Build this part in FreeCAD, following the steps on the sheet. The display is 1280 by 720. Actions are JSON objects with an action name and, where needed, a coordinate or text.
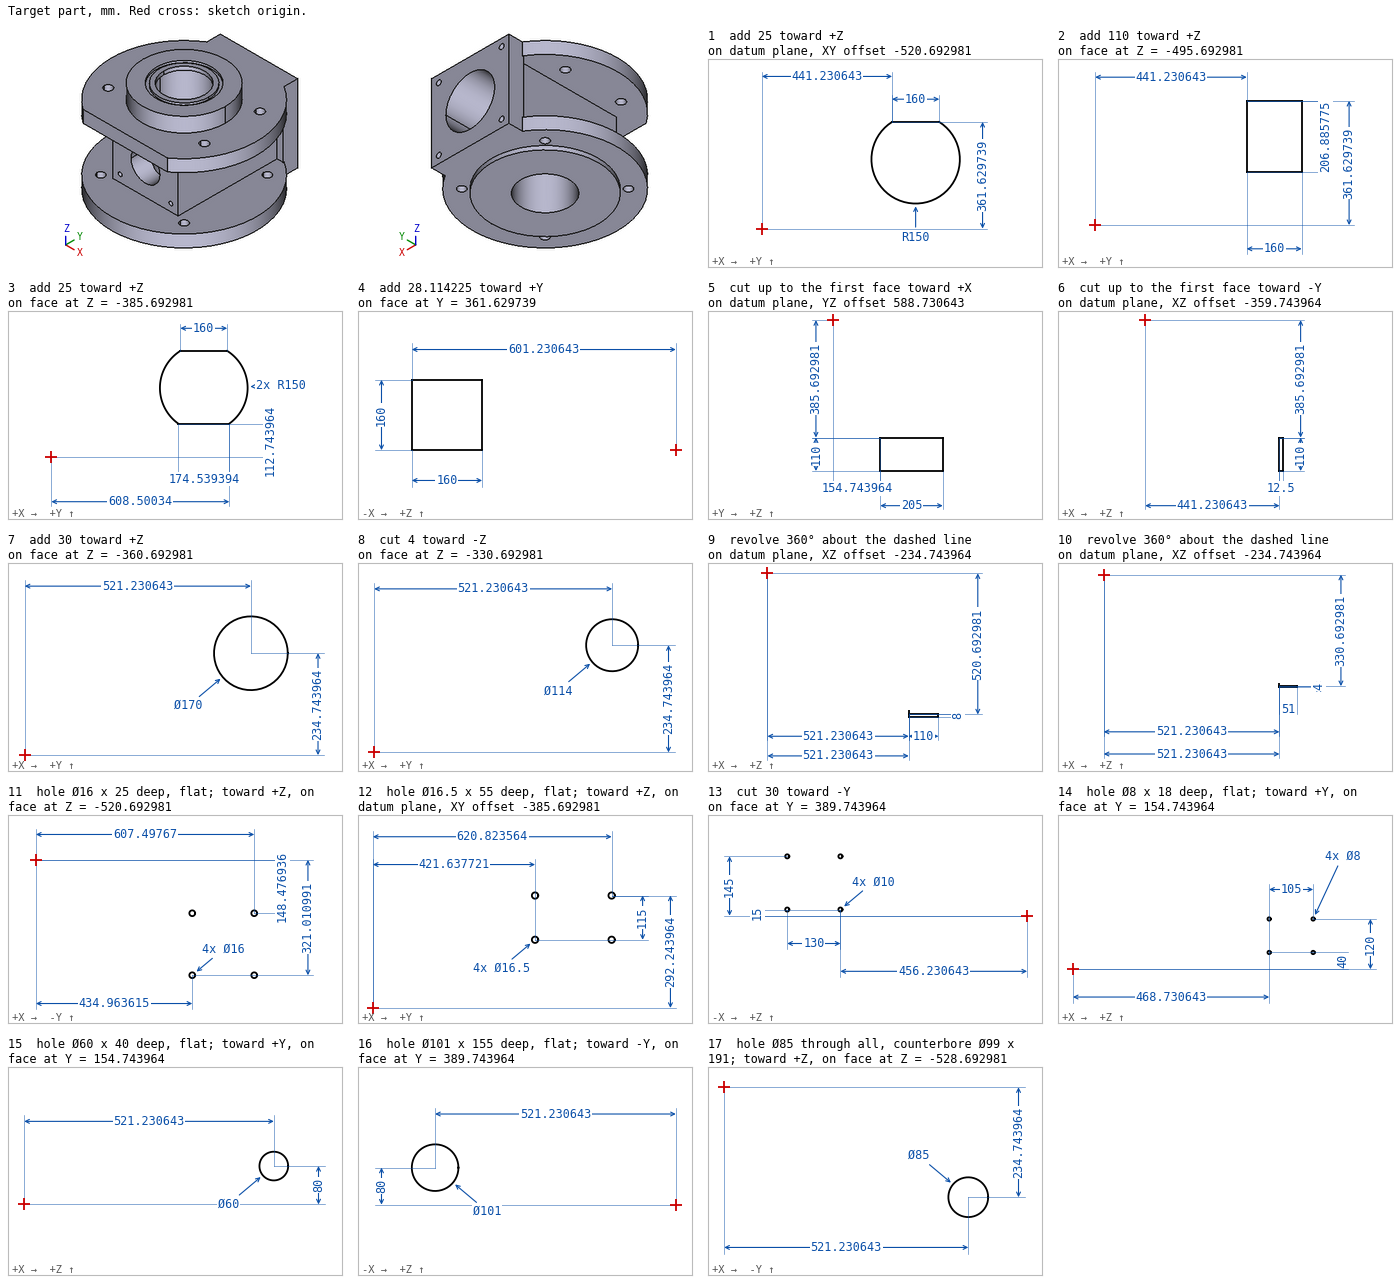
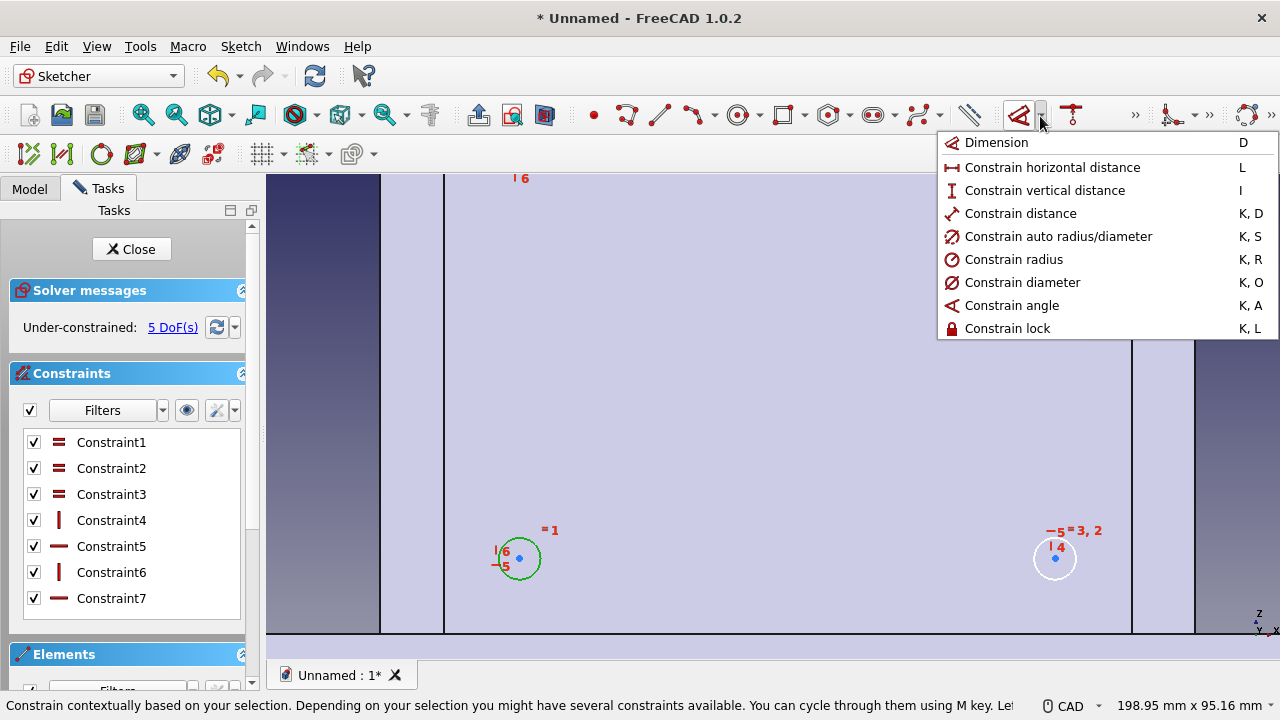
{"action": "left_click", "coordinate": [1108, 282]}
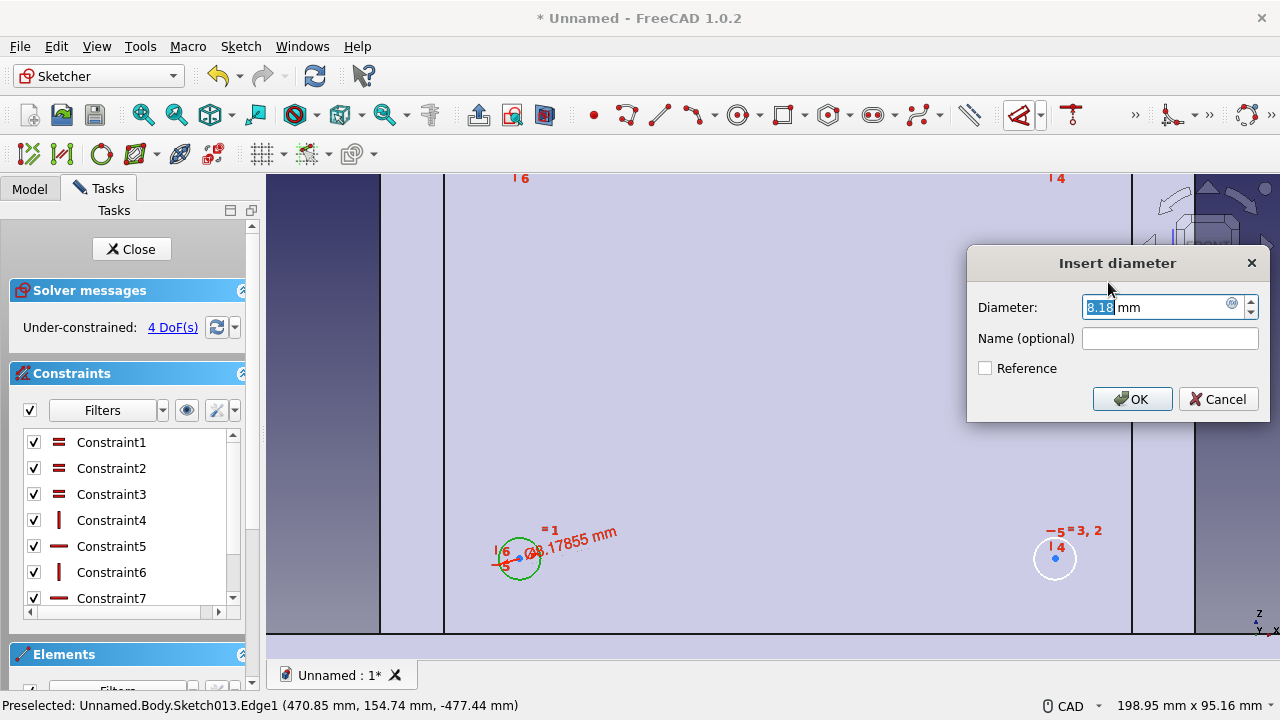
{"action": "type", "text": "8"}
{"action": "key", "text": "Return"}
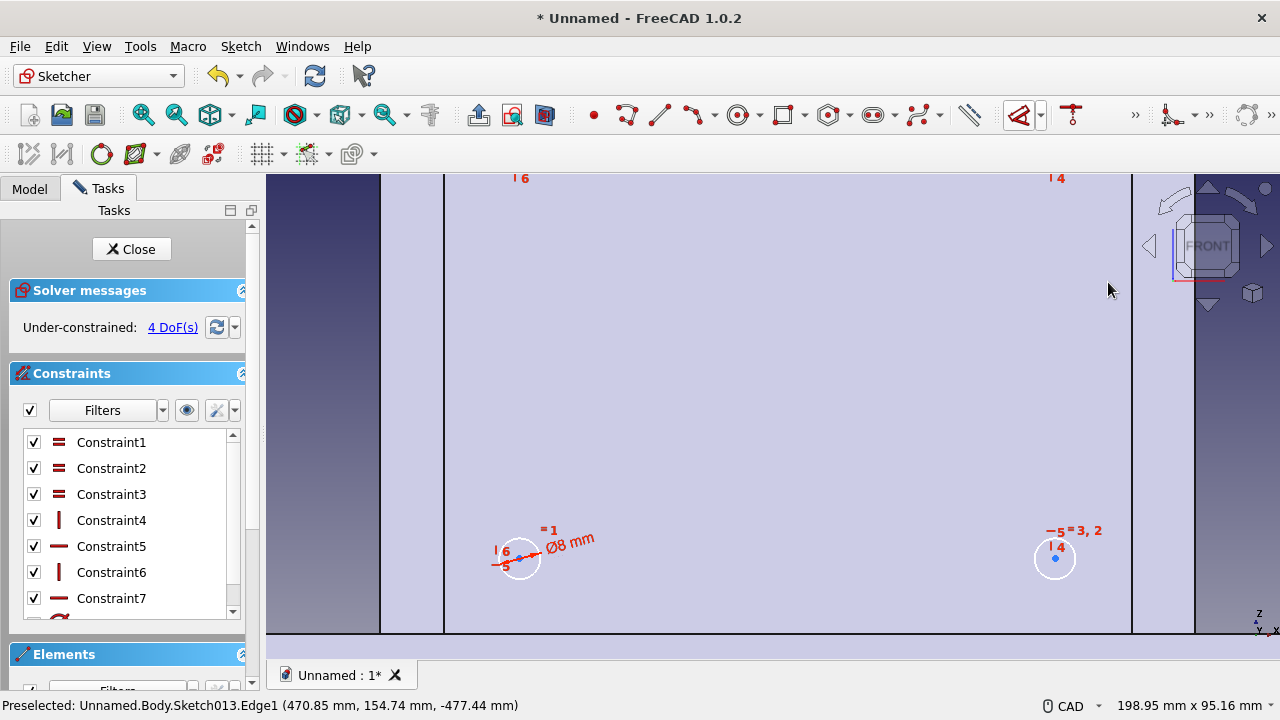
{"action": "left_click", "coordinate": [520, 559]}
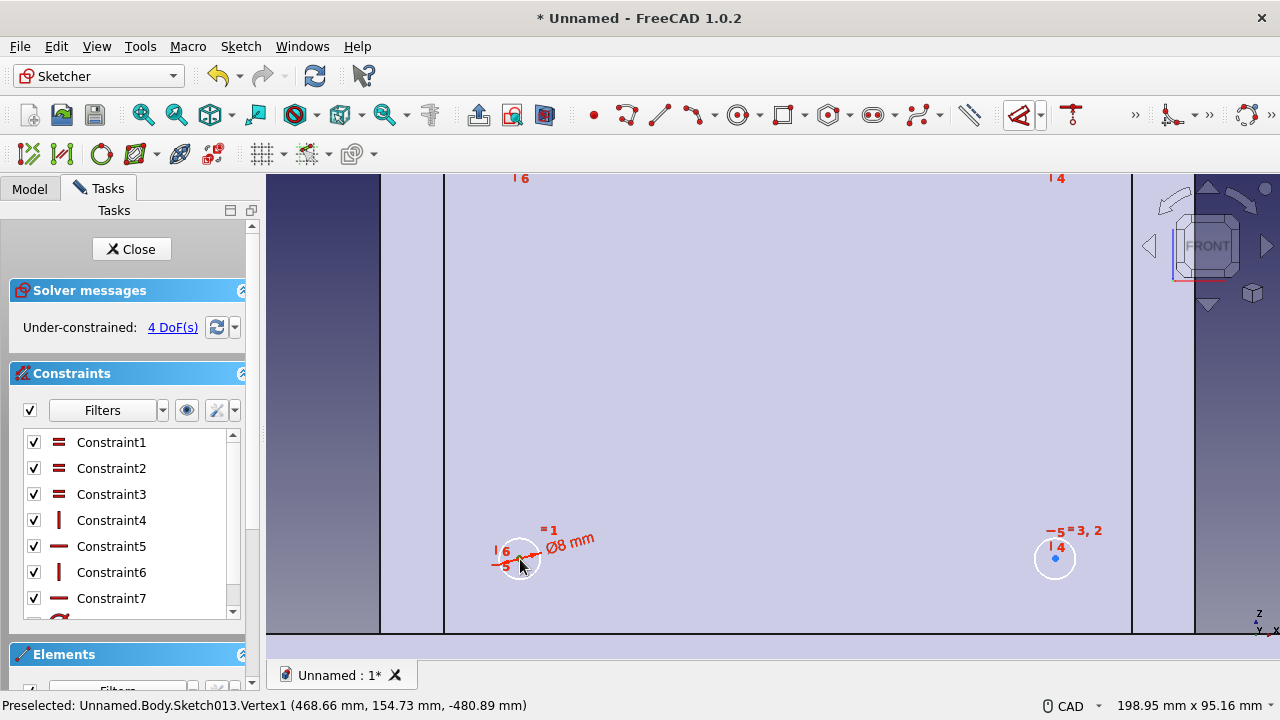
{"action": "key", "text": "i"}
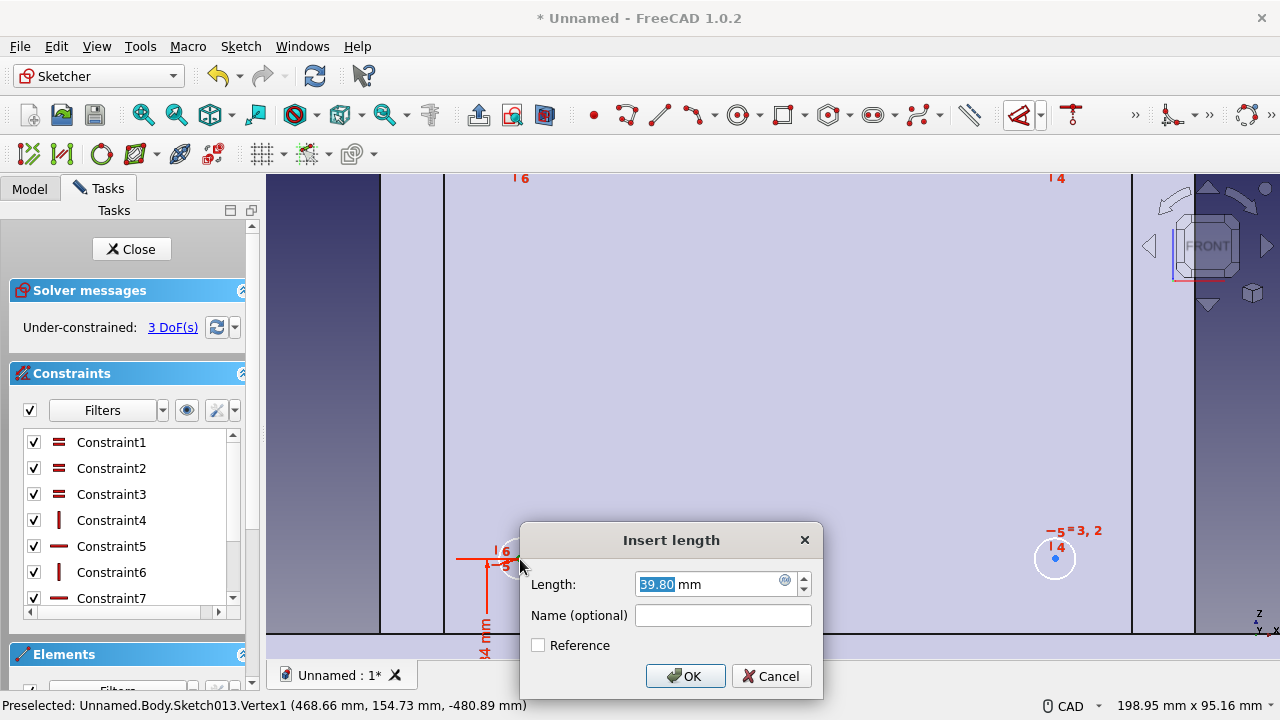
{"action": "type", "text": "40"}
{"action": "key", "text": "Return"}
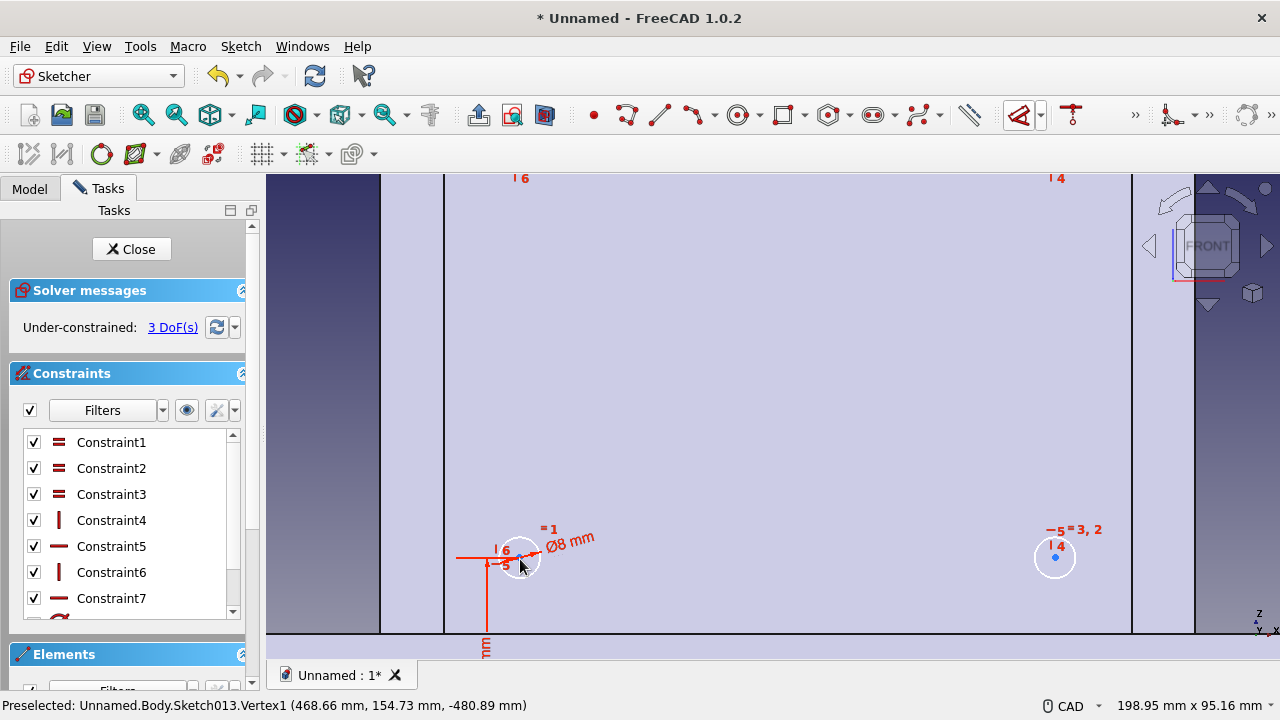
{"action": "scroll", "coordinate": [535, 544], "scroll_direction": "down", "scroll_amount": 2}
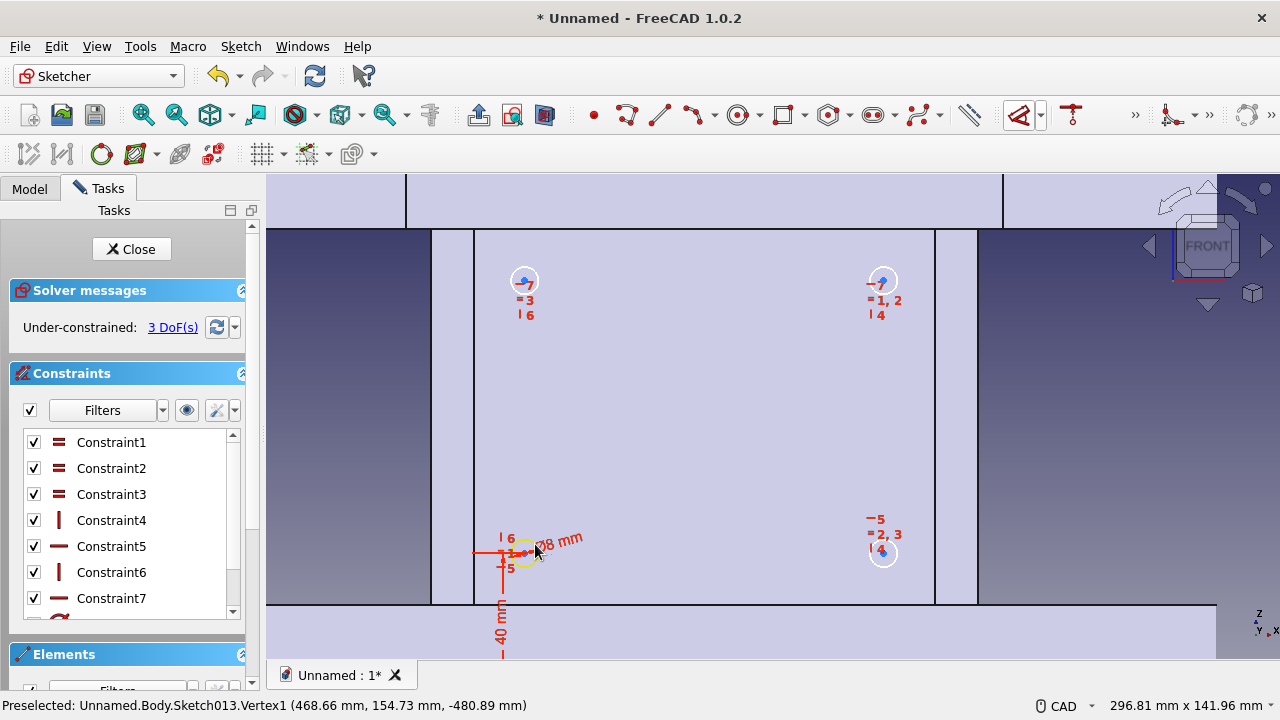
{"action": "left_click", "coordinate": [884, 281]}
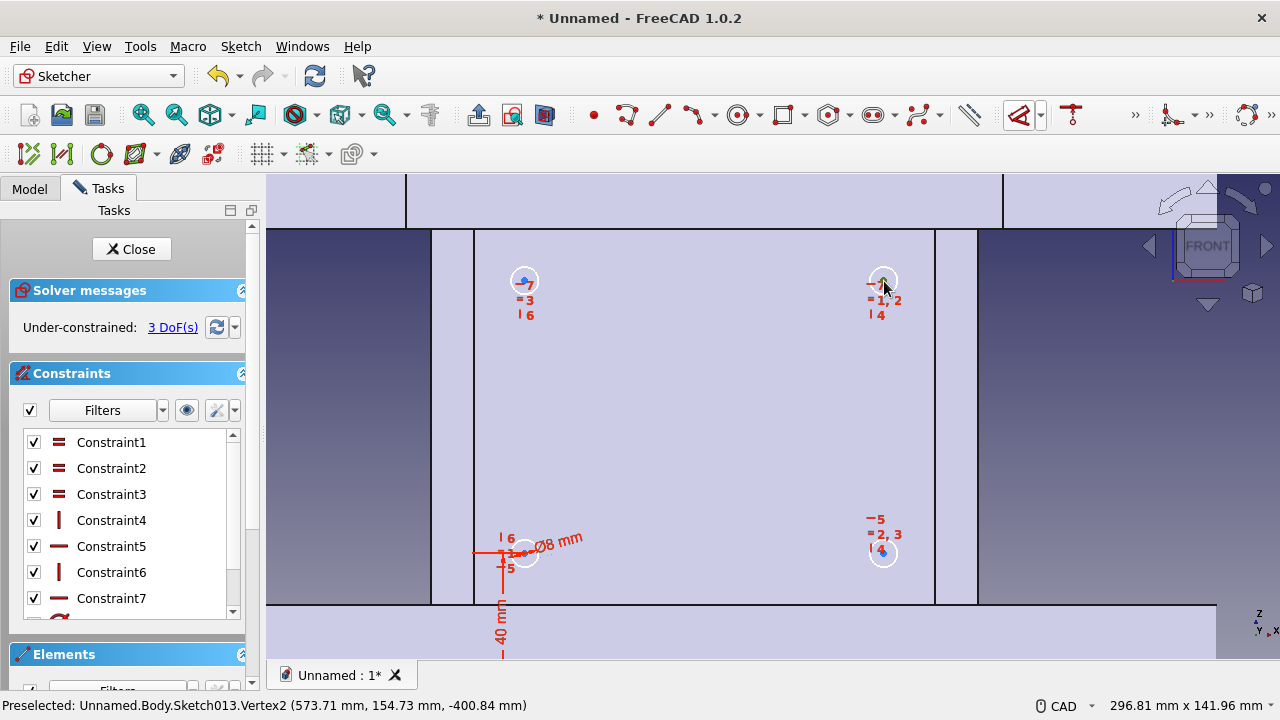
{"action": "left_click", "coordinate": [1040, 116]}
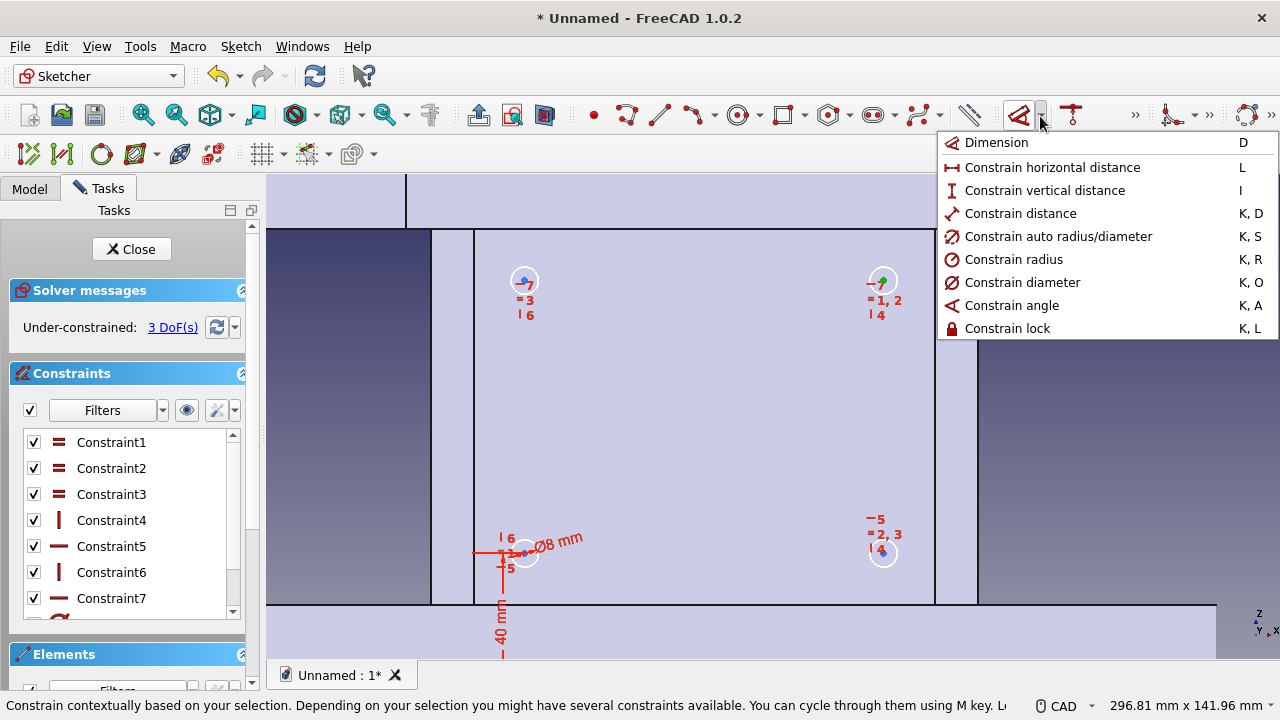
{"action": "left_click", "coordinate": [1108, 190]}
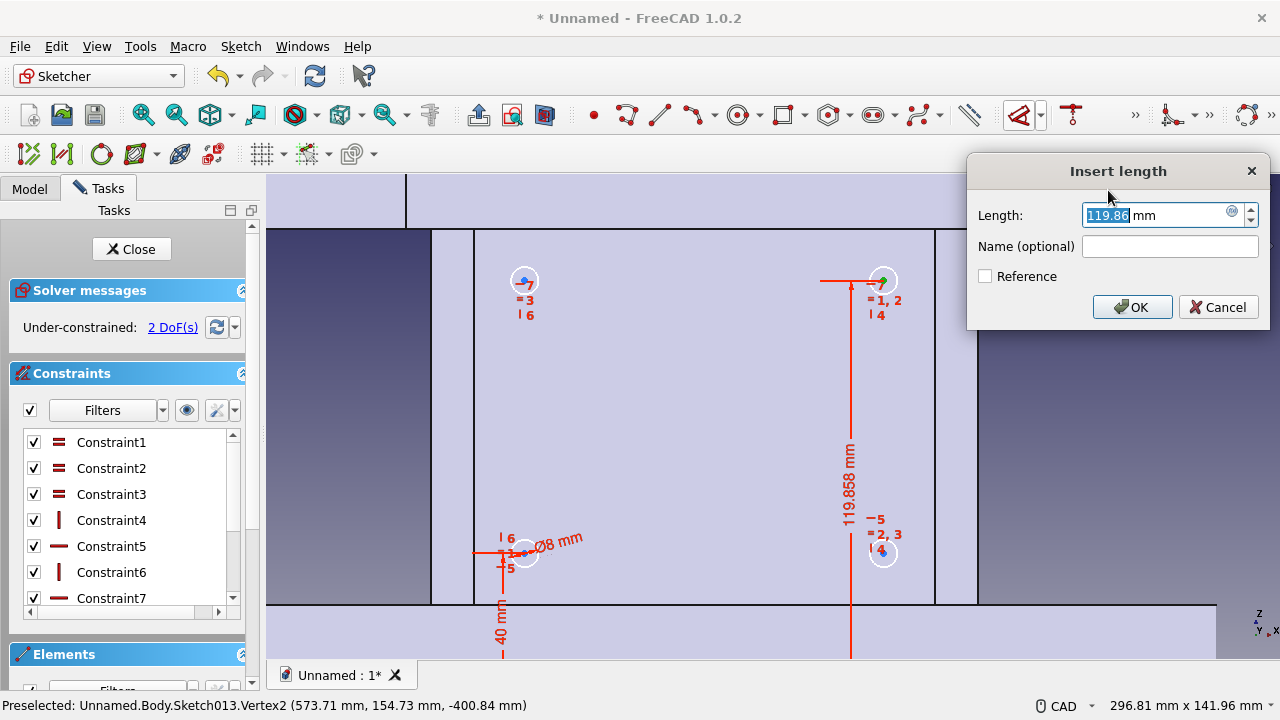
{"action": "type", "text": "120"}
{"action": "key", "text": "Return"}